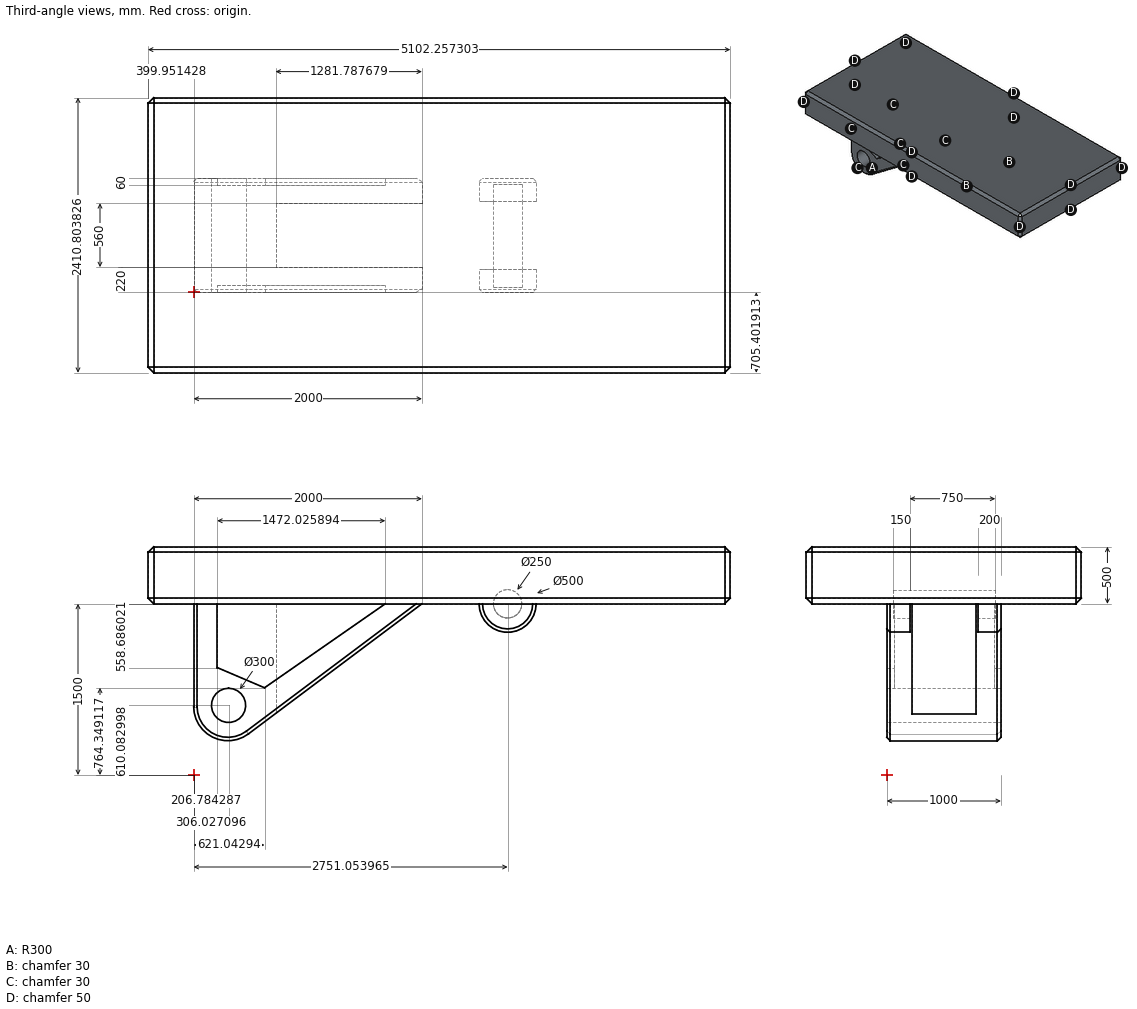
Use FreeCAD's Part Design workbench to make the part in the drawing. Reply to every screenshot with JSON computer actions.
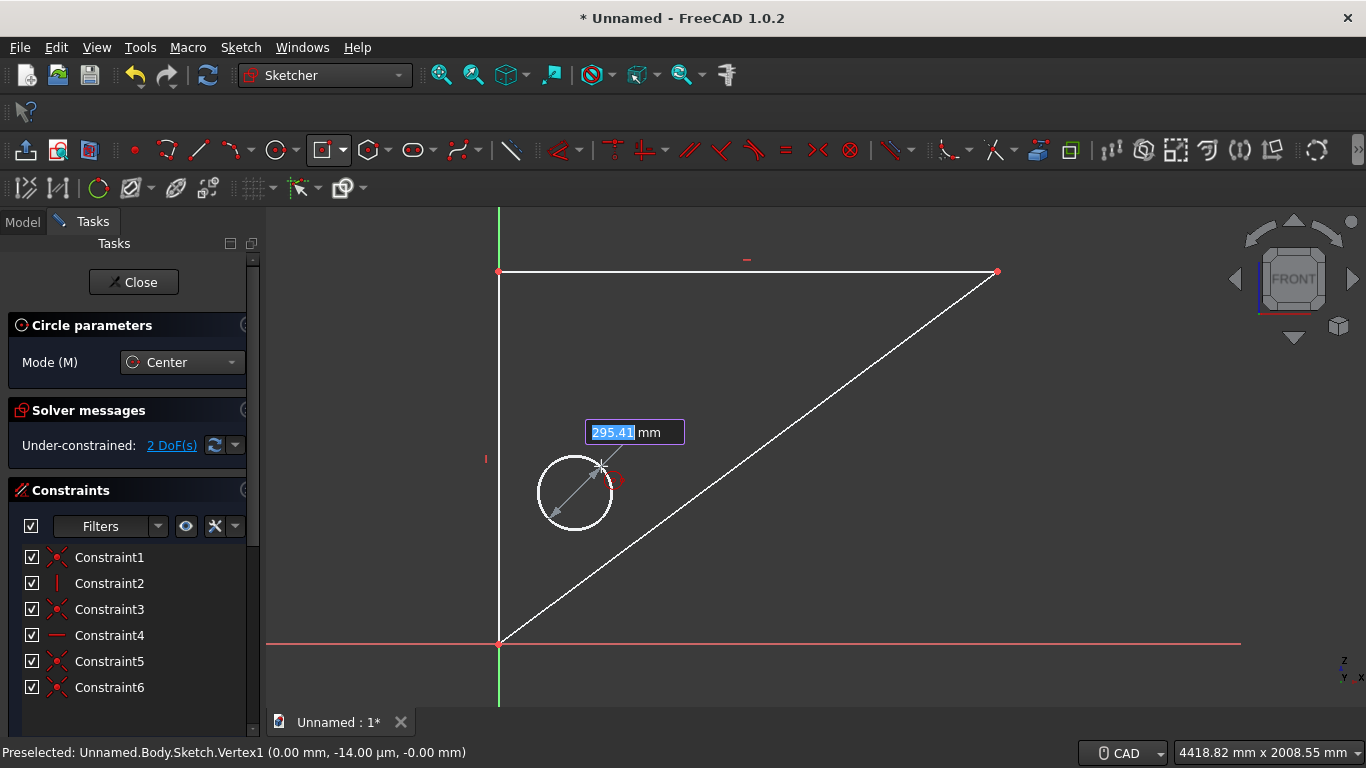
{"action": "type", "text": "300"}
{"action": "key", "text": "Return"}
{"action": "key", "text": "Escape"}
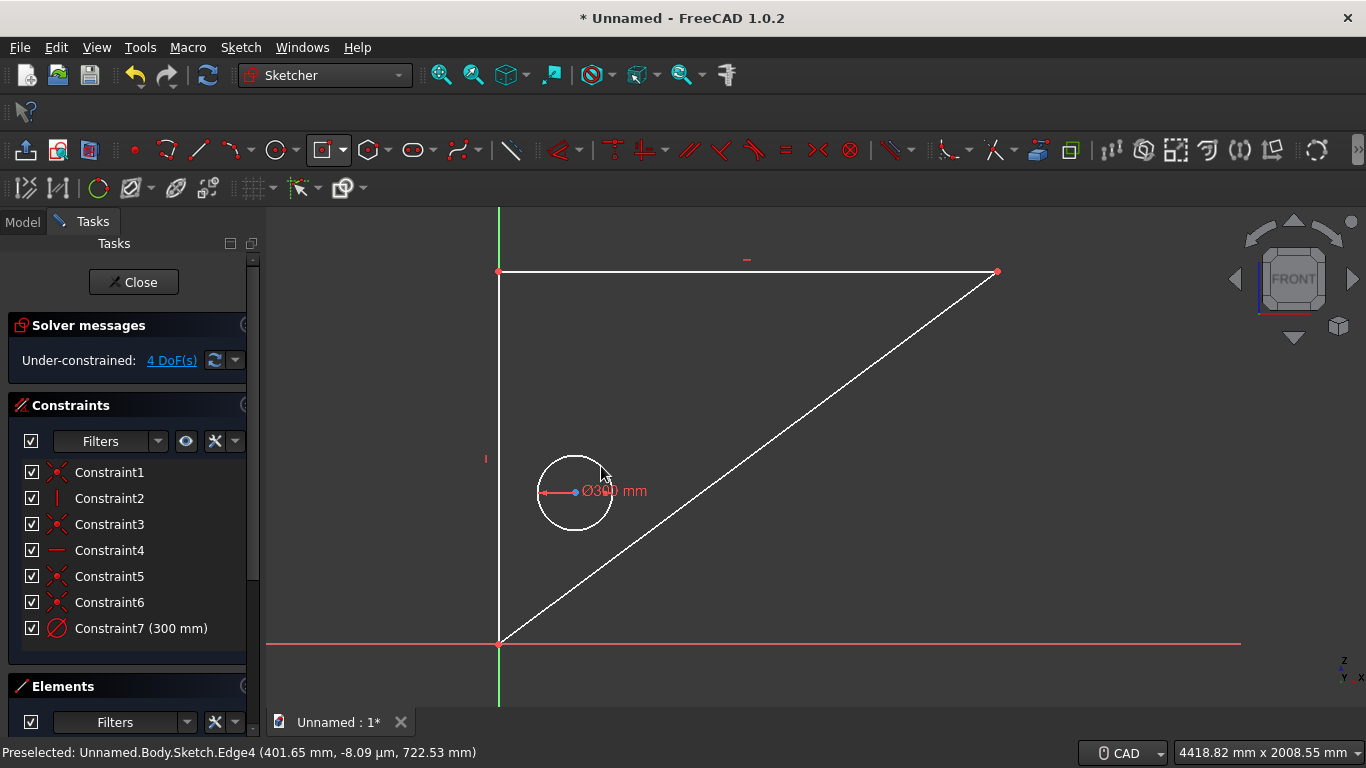
{"action": "key", "text": "d"}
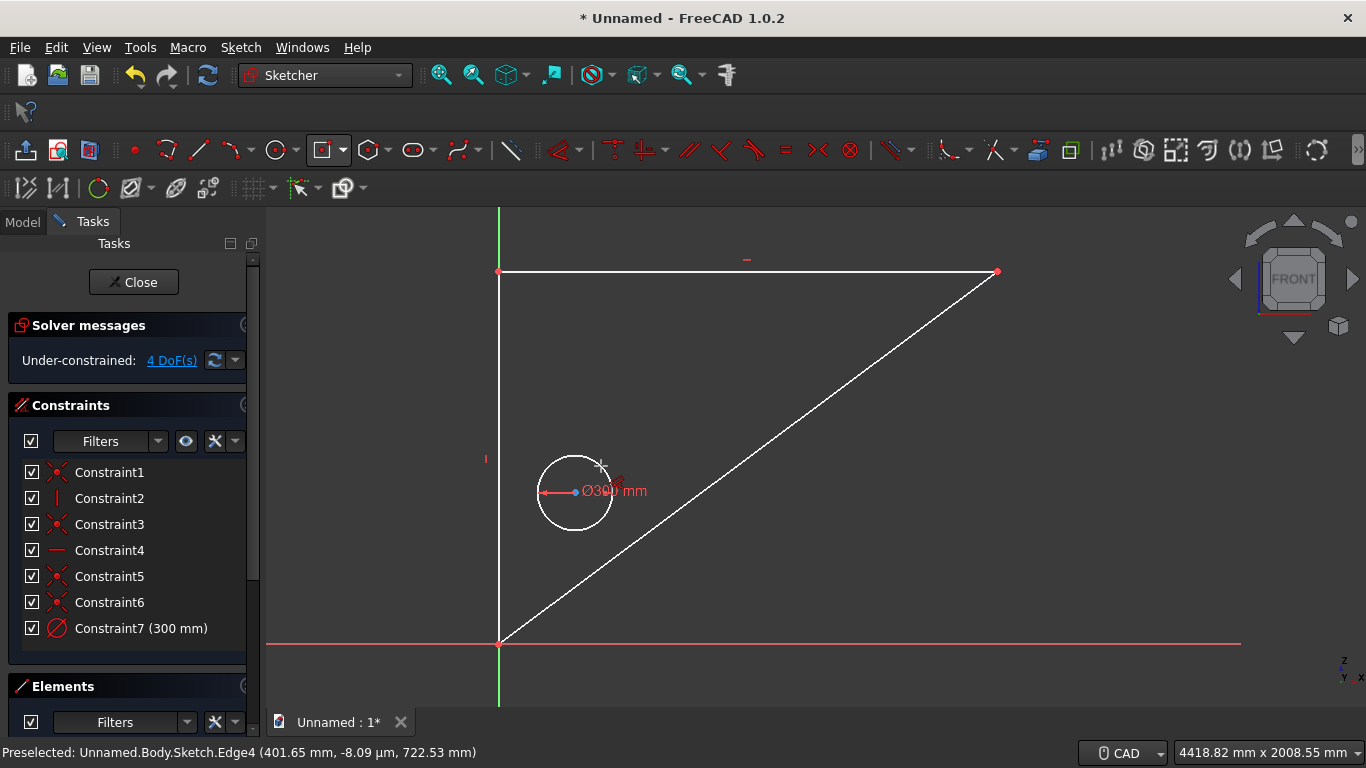
{"action": "left_click", "coordinate": [499, 532]}
{"action": "left_click", "coordinate": [465, 458]}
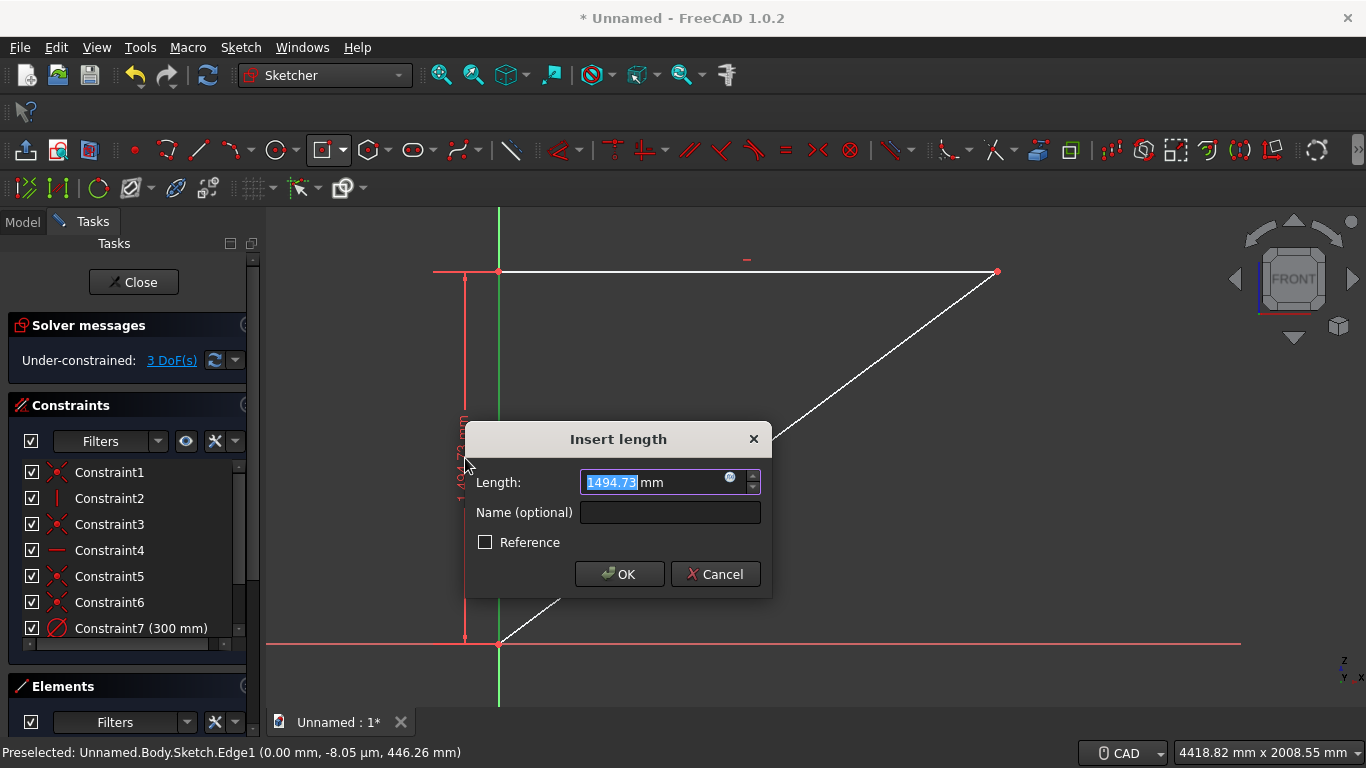
{"action": "type", "text": "1500"}
{"action": "key", "text": "Return"}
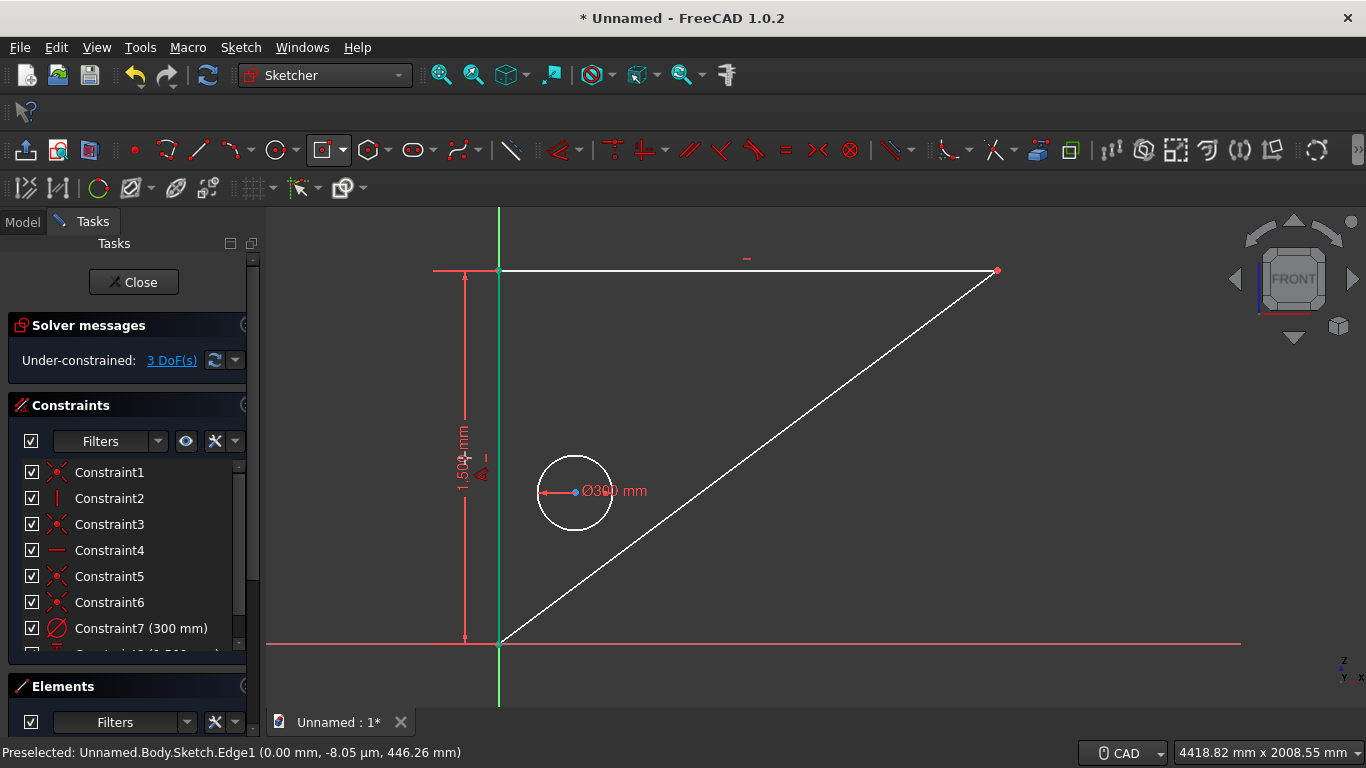
{"action": "left_click", "coordinate": [648, 271]}
{"action": "left_click", "coordinate": [748, 237]}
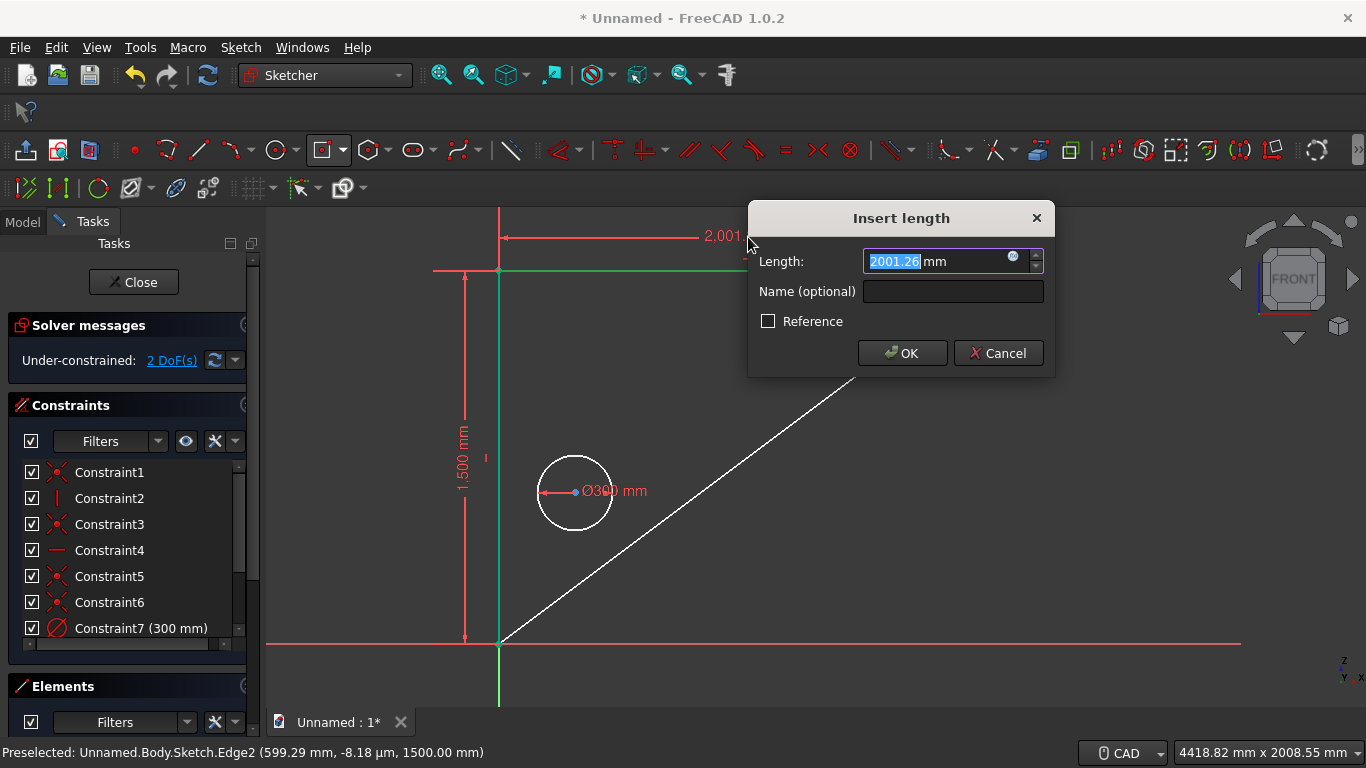
{"action": "type", "text": "2000"}
{"action": "key", "text": "Return"}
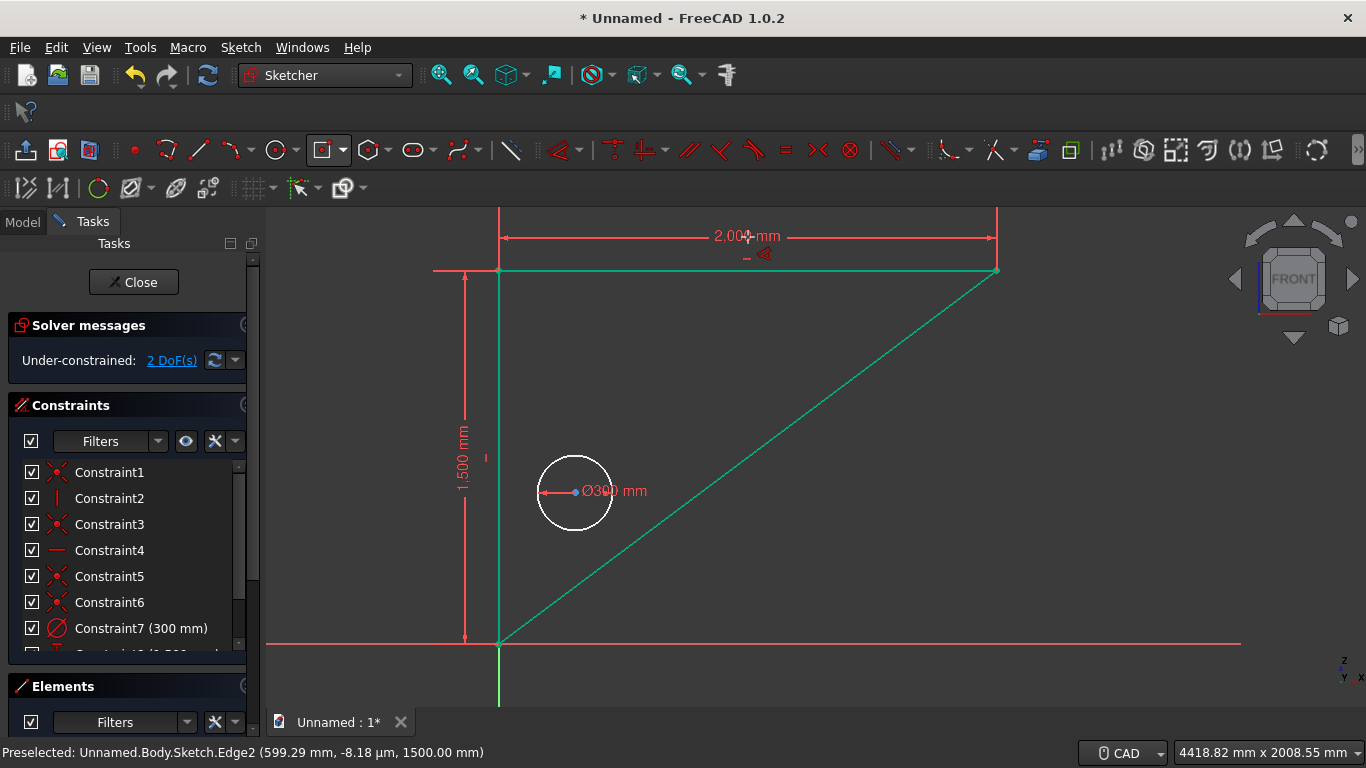
{"action": "left_click", "coordinate": [575, 493]}
{"action": "left_click", "coordinate": [537, 678]}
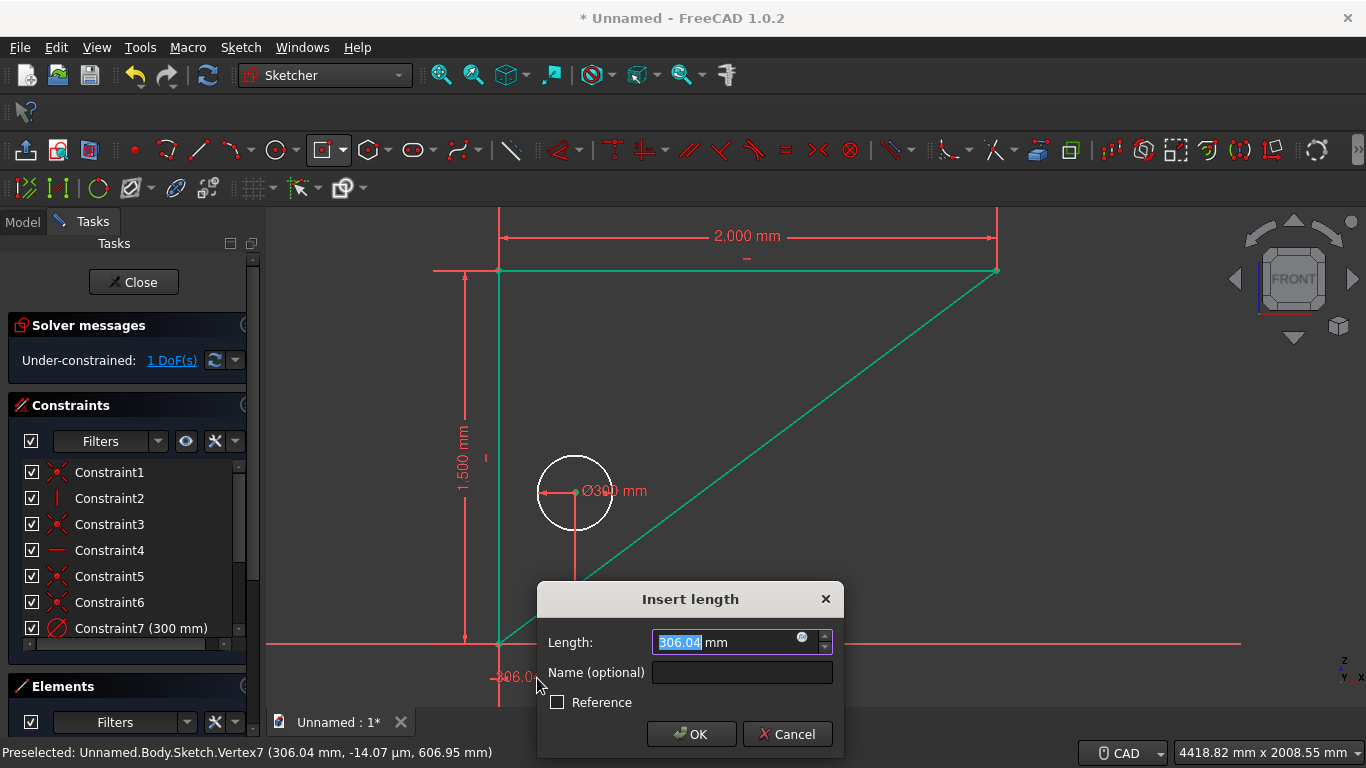
{"action": "type", "text": "306.027096"}
{"action": "key", "text": "Return"}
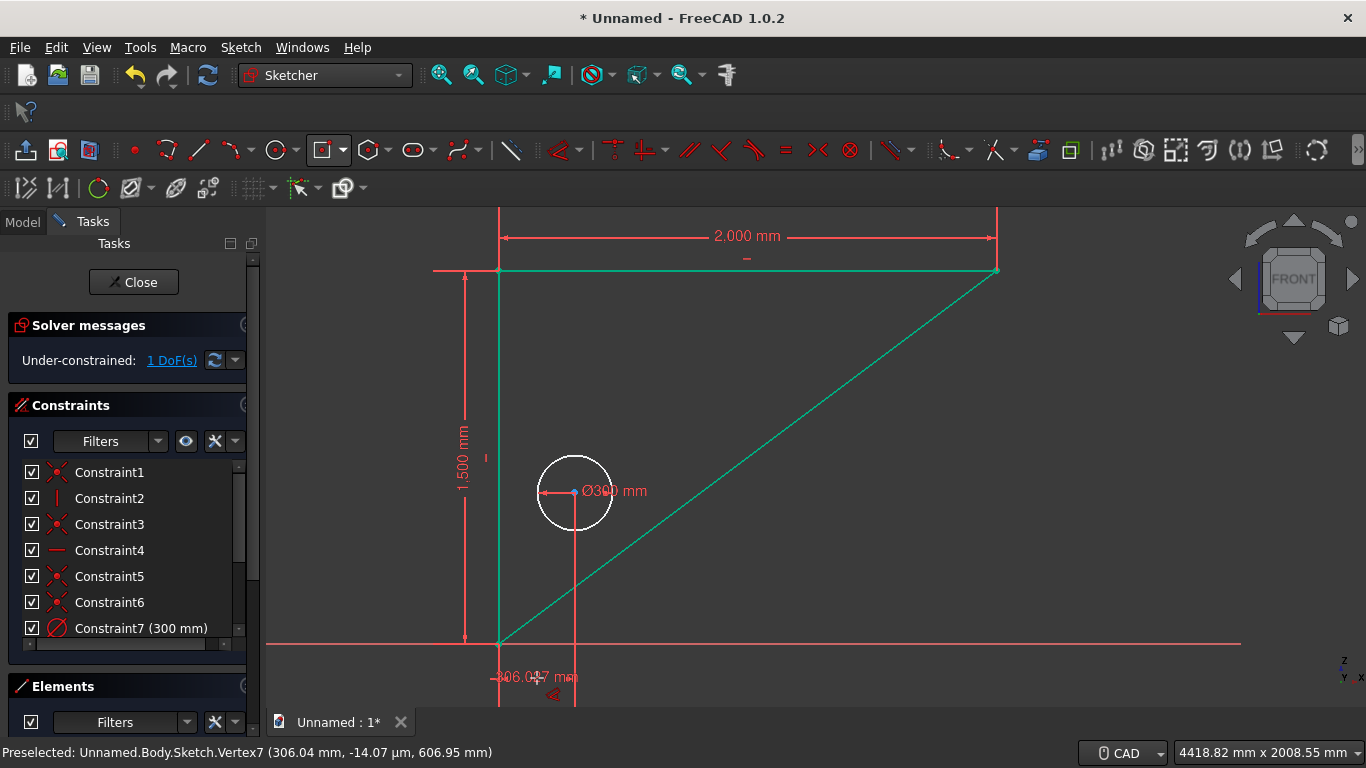
{"action": "left_click", "coordinate": [575, 493]}
{"action": "left_click", "coordinate": [465, 569]}